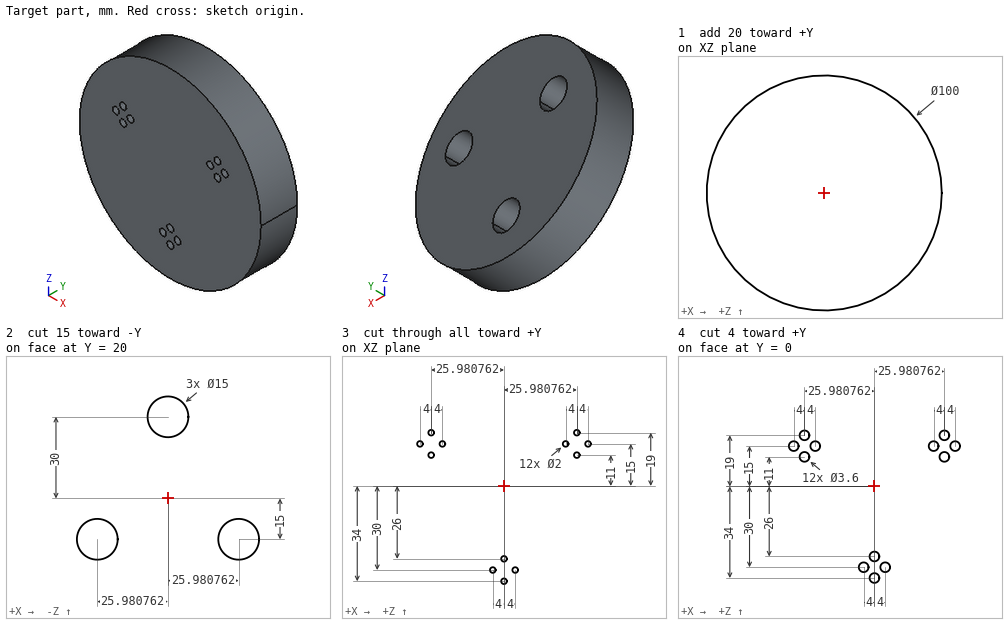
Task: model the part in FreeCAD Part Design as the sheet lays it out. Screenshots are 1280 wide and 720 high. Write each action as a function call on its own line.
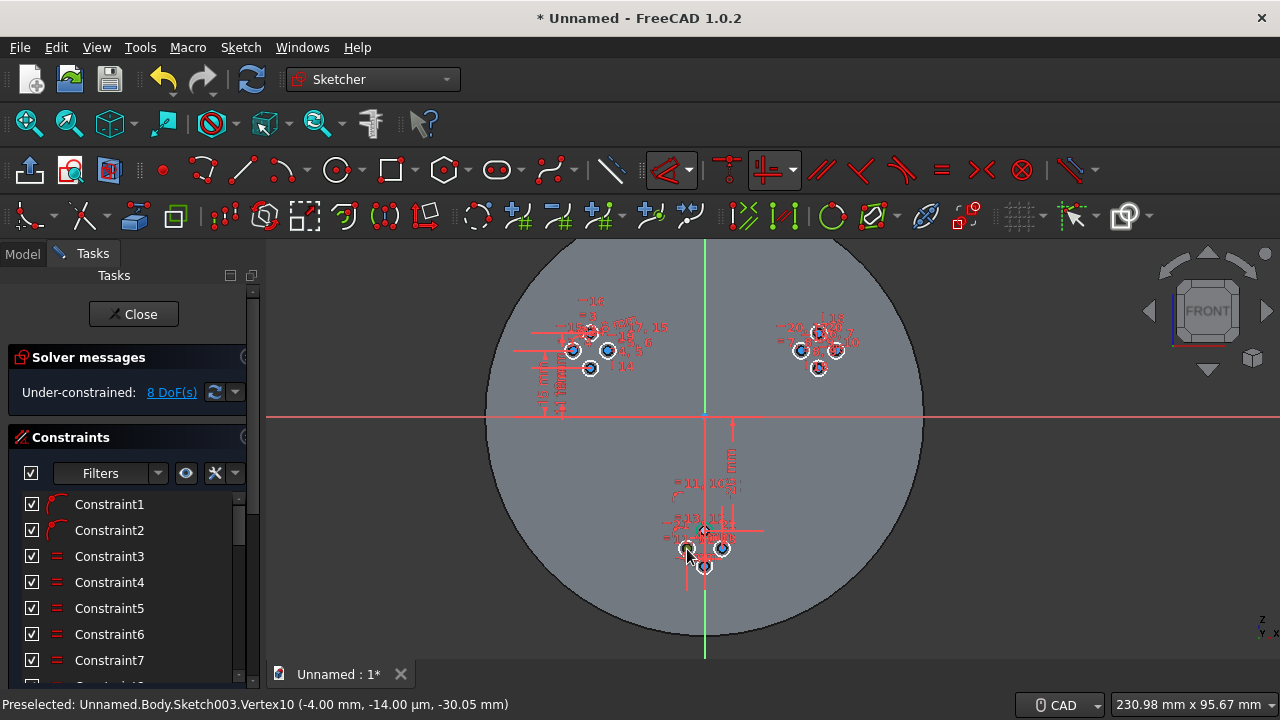
click(692, 170)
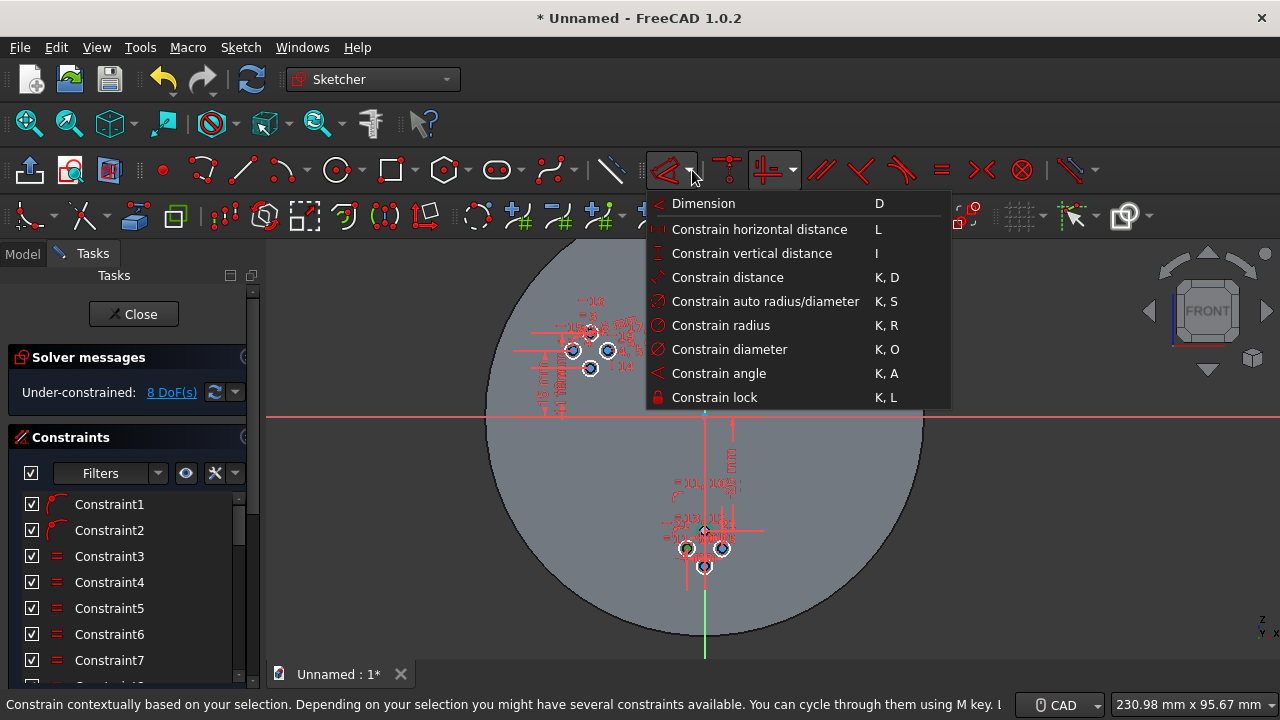
click(799, 253)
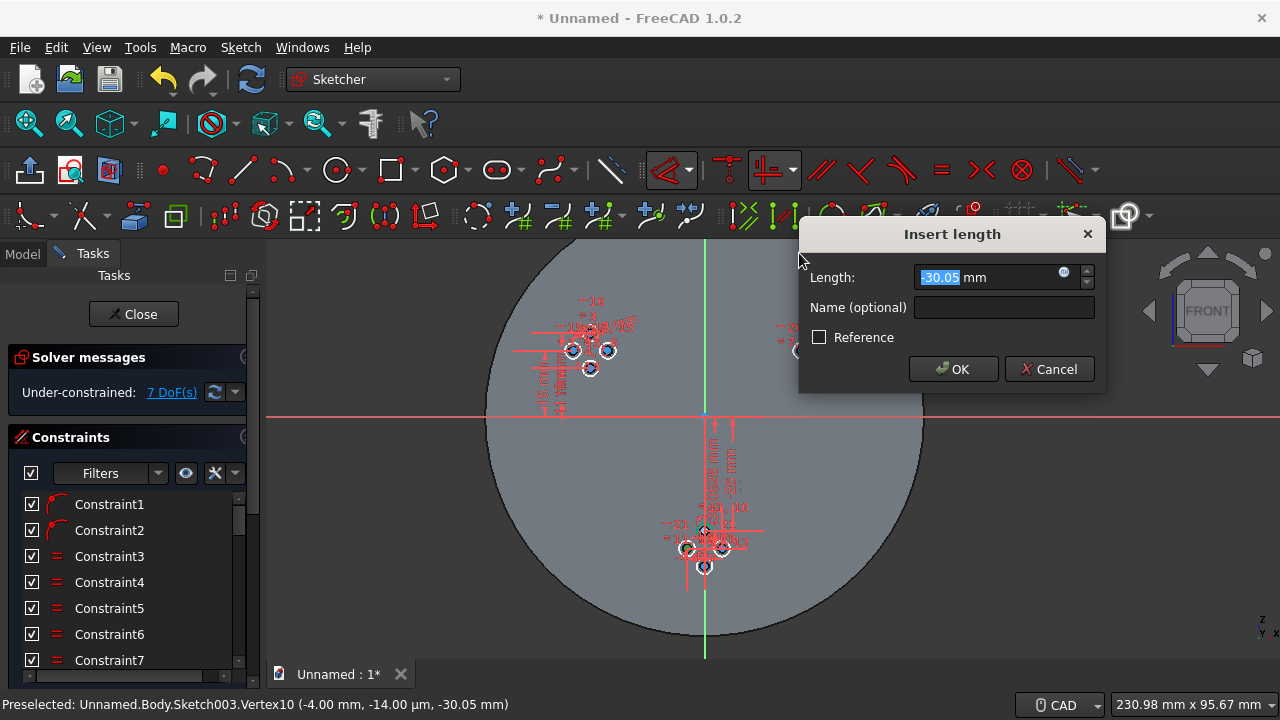
text(-30)
key(Return)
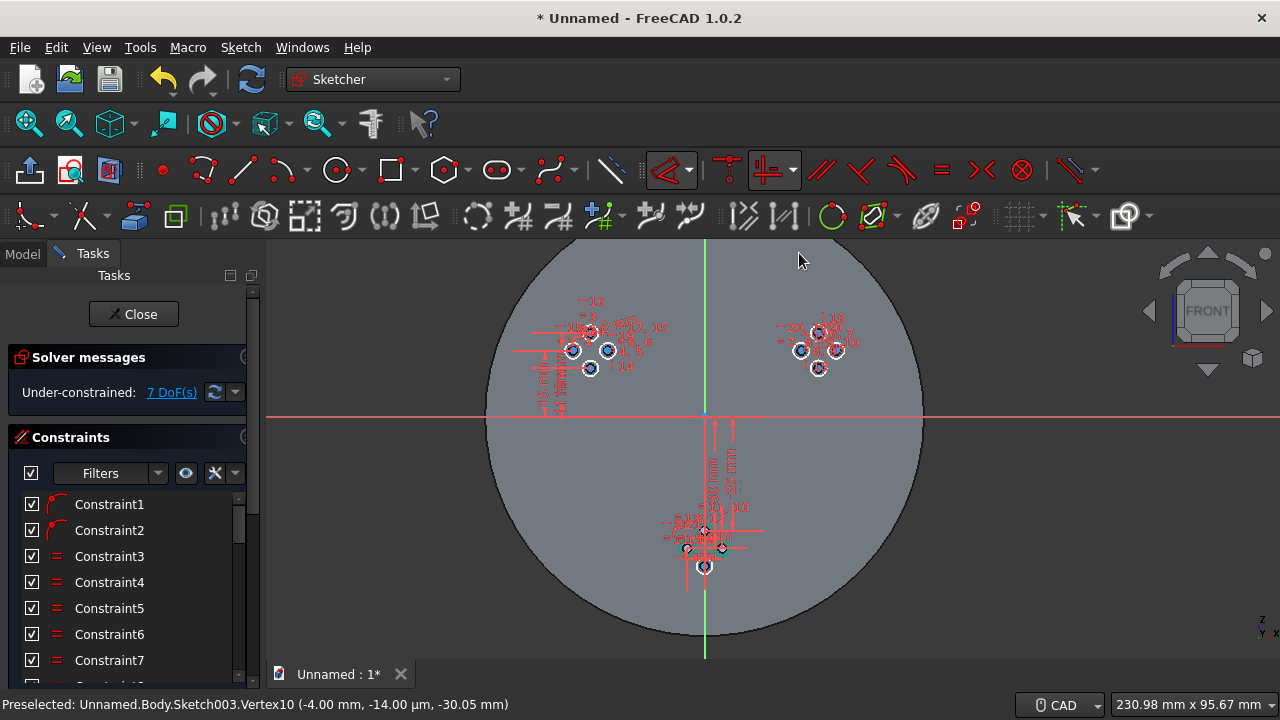
click(705, 566)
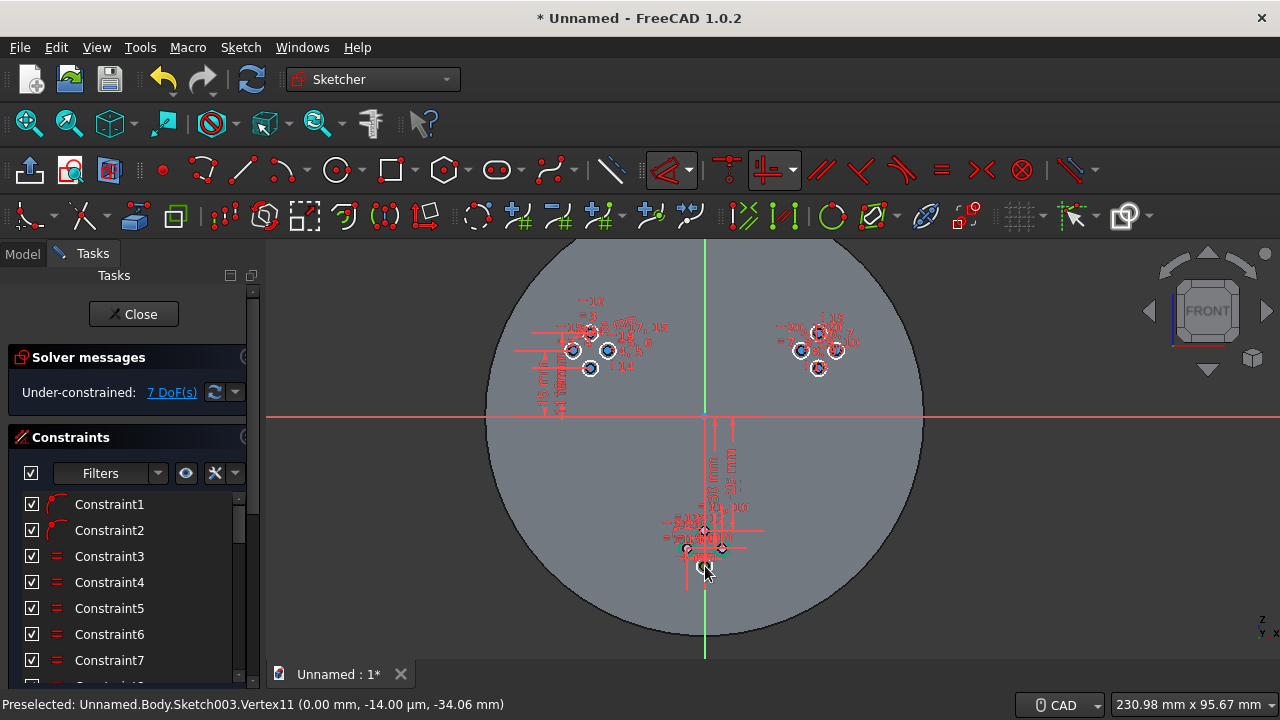
key(i)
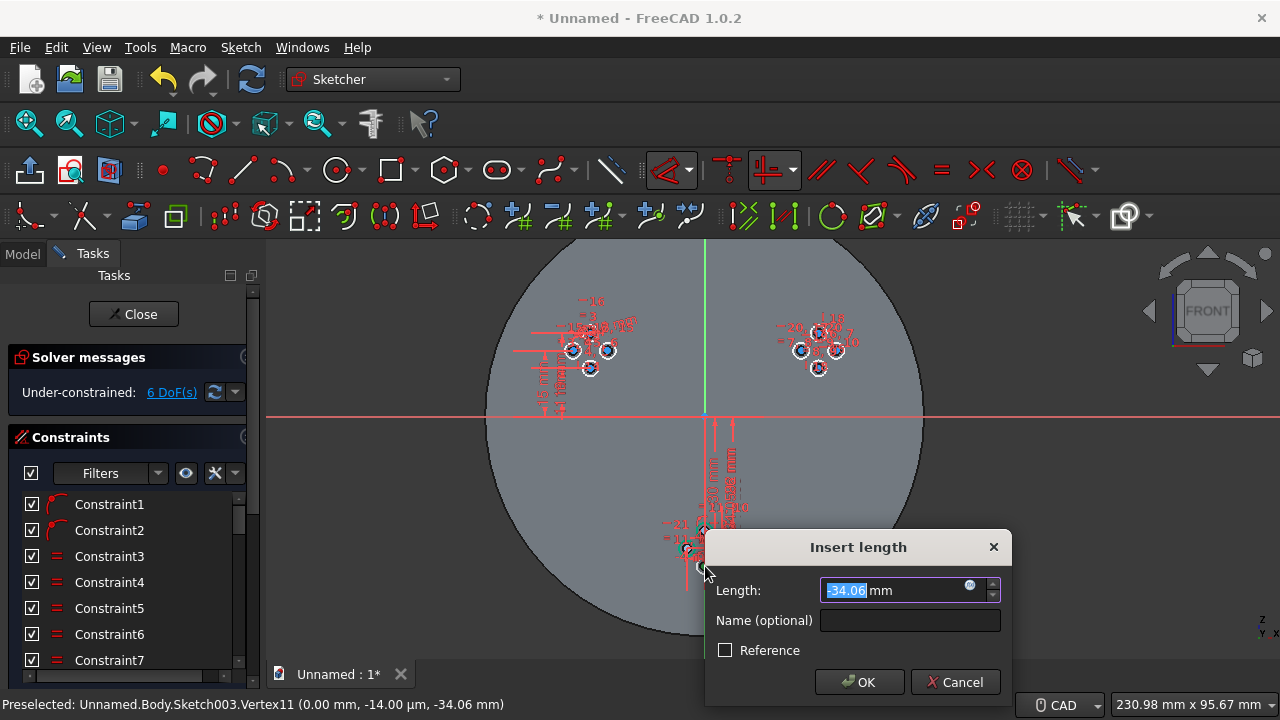
text(-34)
key(Return)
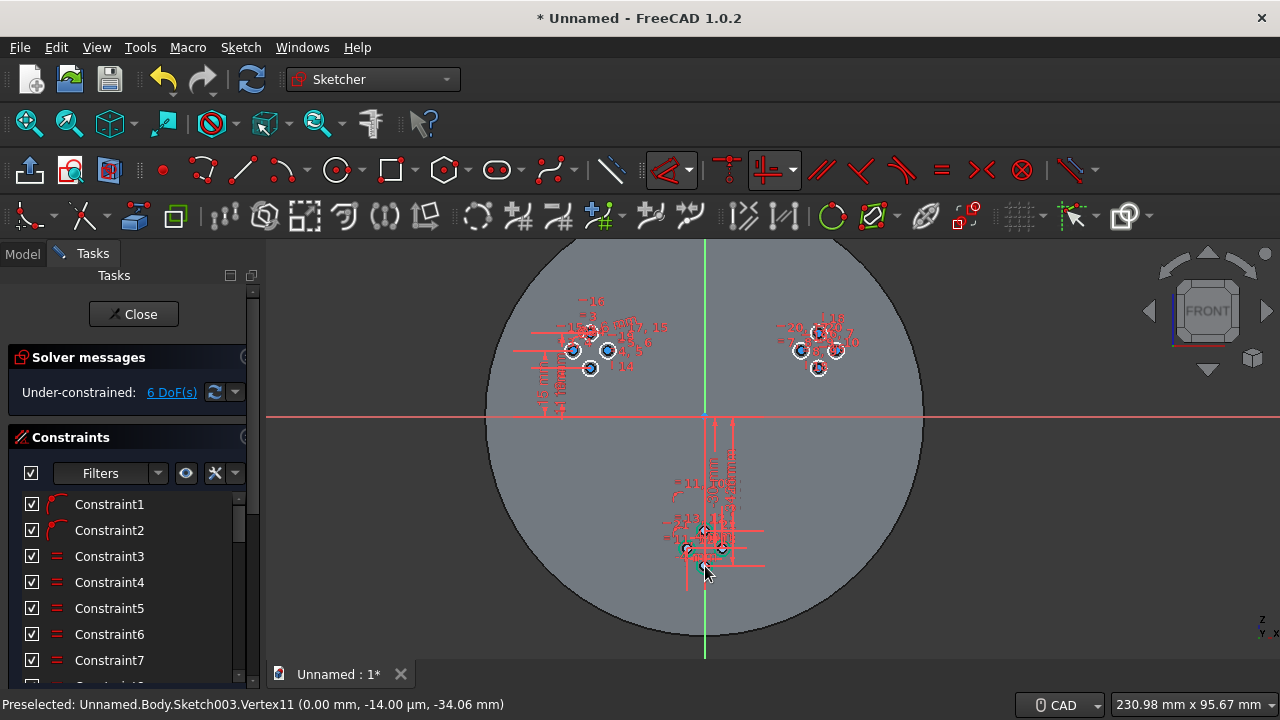
scroll(590, 333, up, 5)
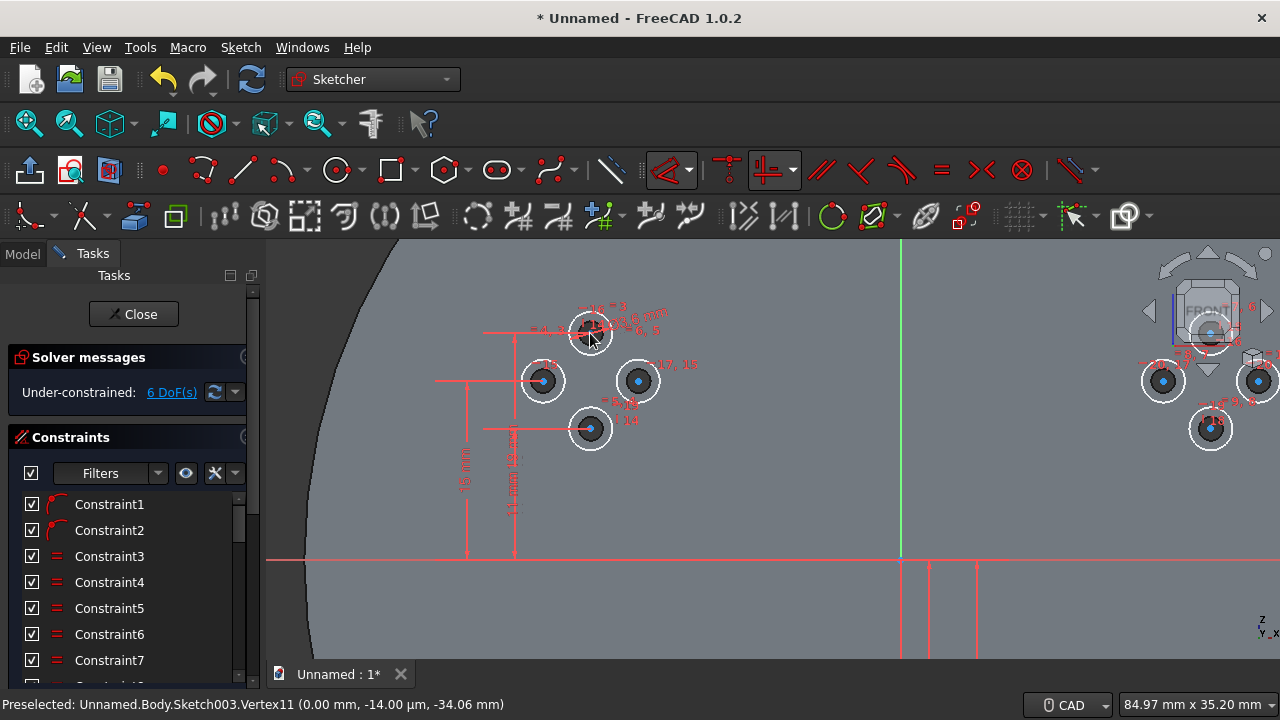
click(591, 333)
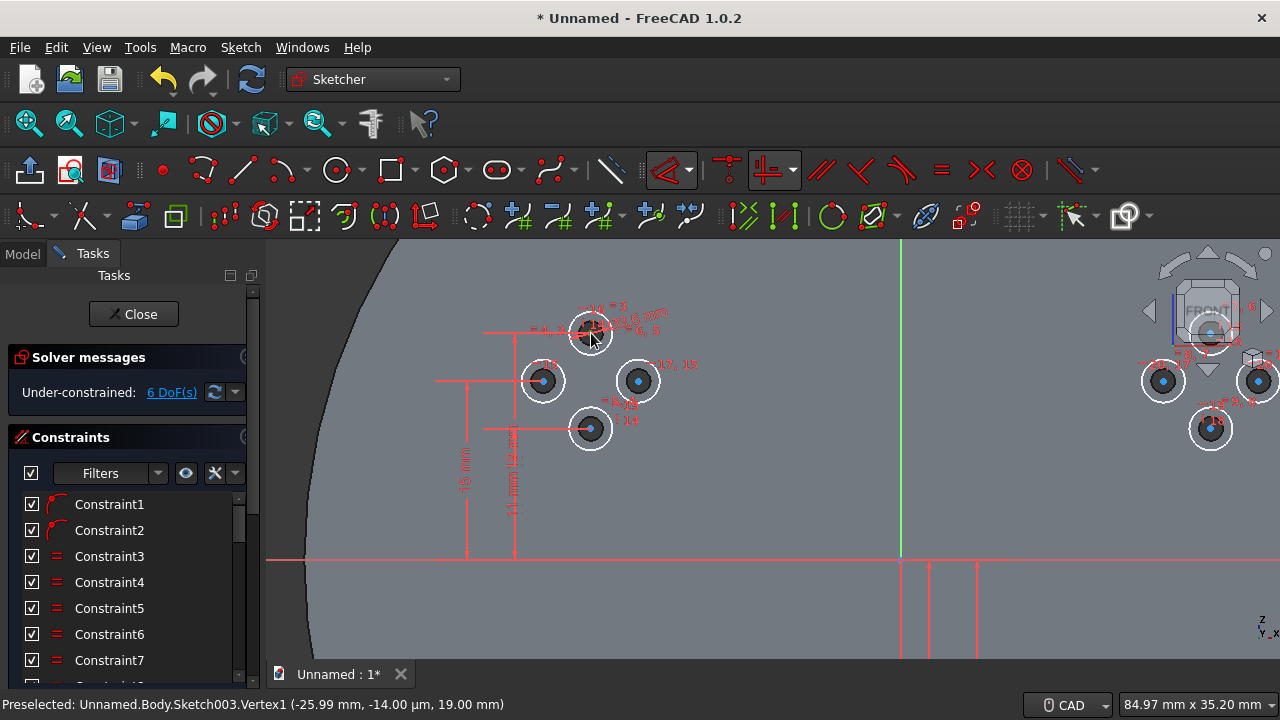
click(543, 381)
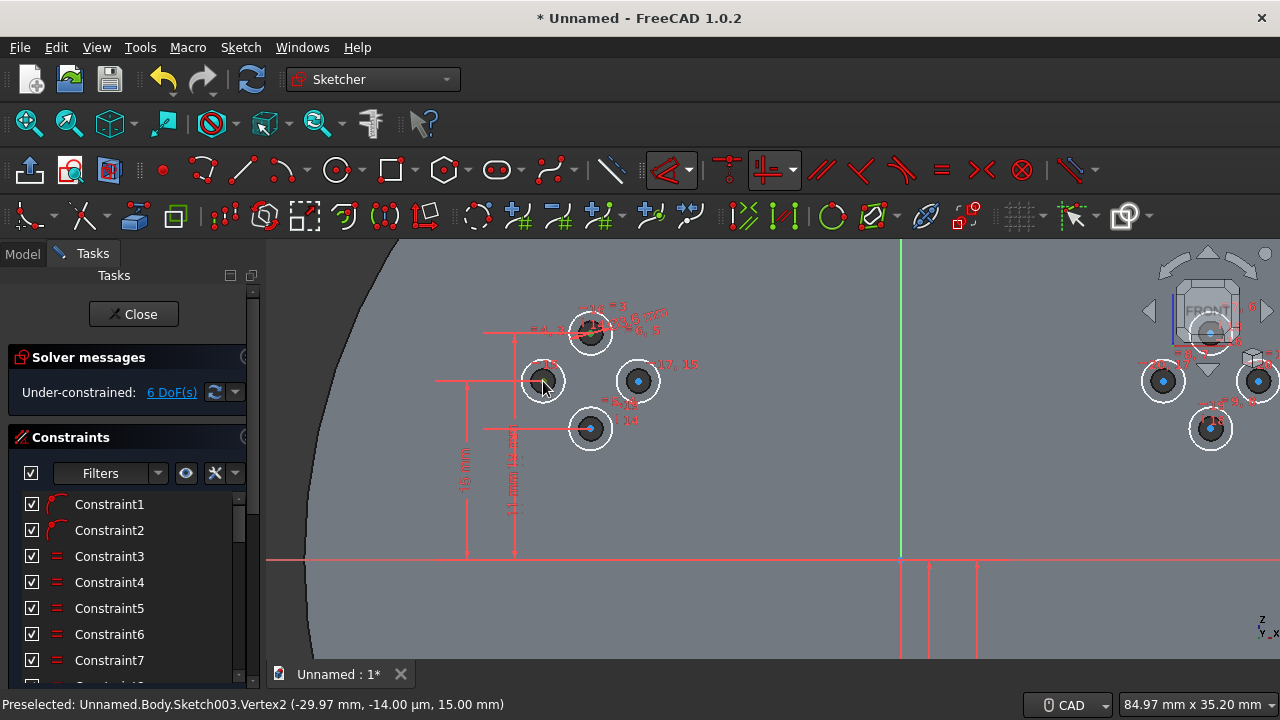
click(692, 170)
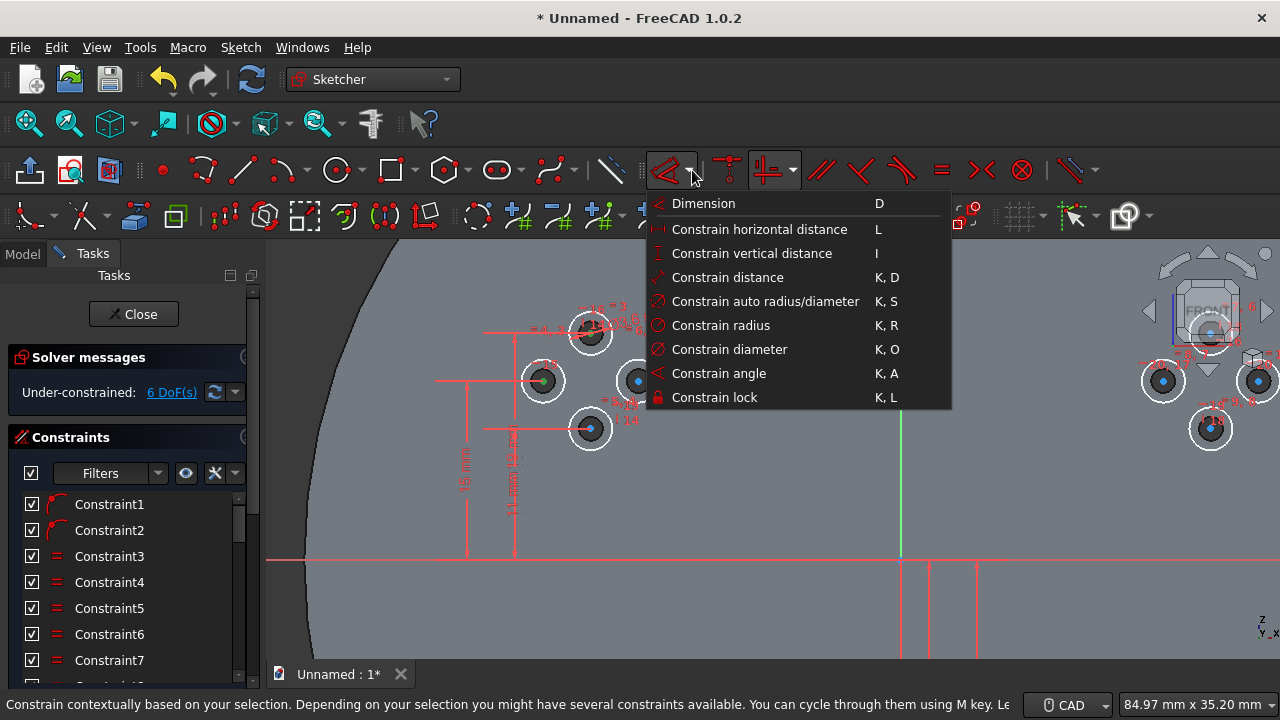
click(799, 229)